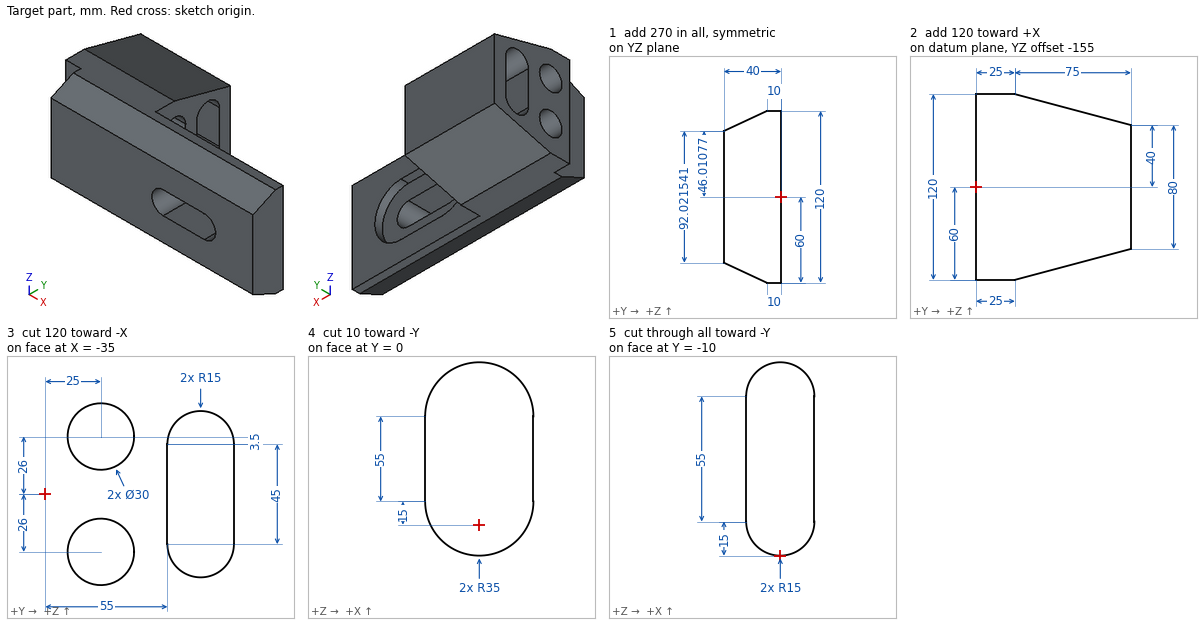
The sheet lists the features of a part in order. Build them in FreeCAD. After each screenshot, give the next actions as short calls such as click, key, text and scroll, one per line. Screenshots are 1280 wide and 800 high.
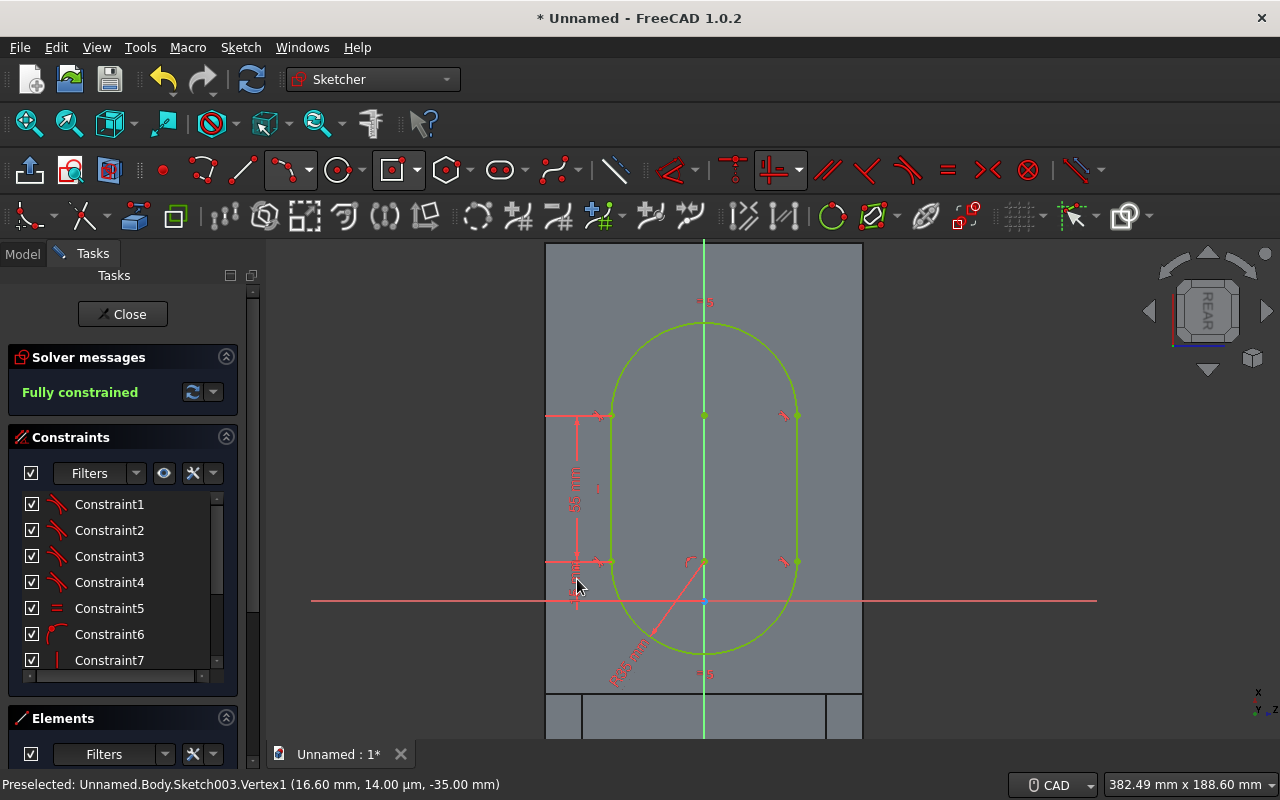
click(123, 314)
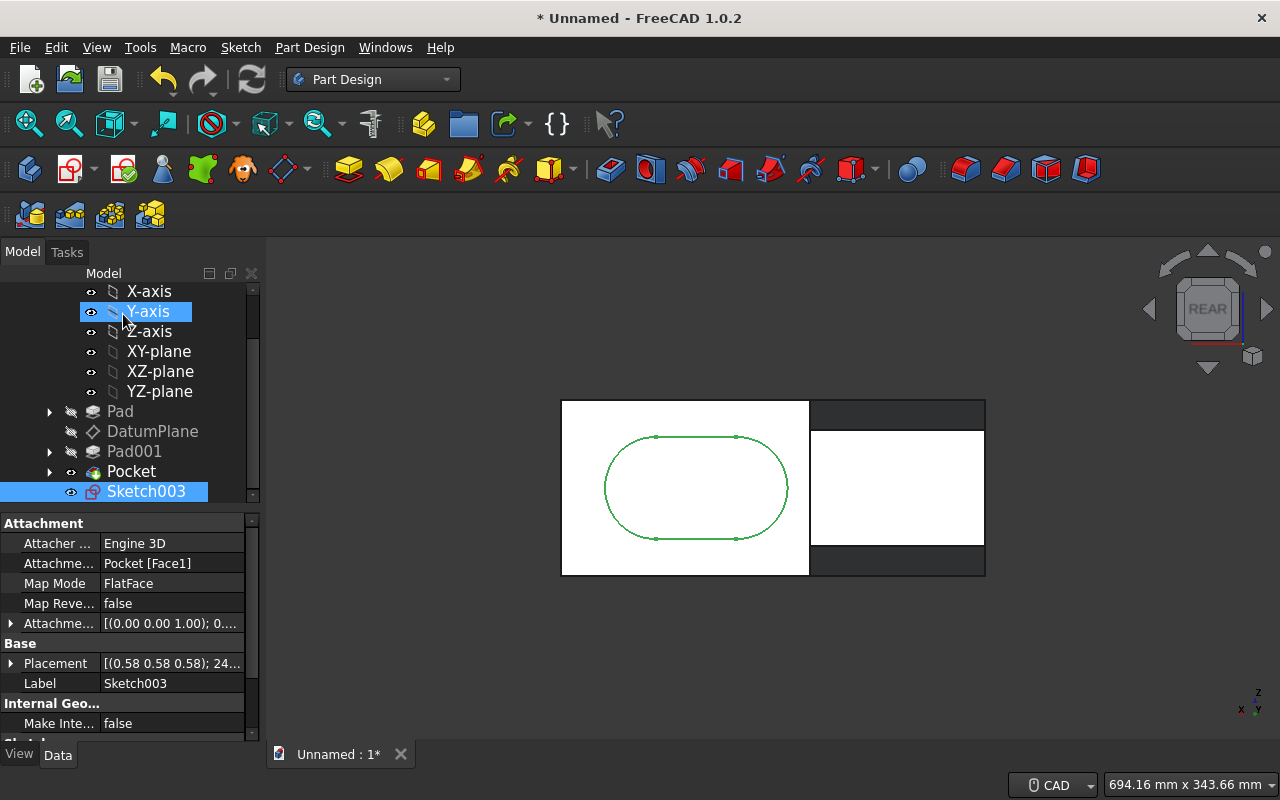
click(612, 170)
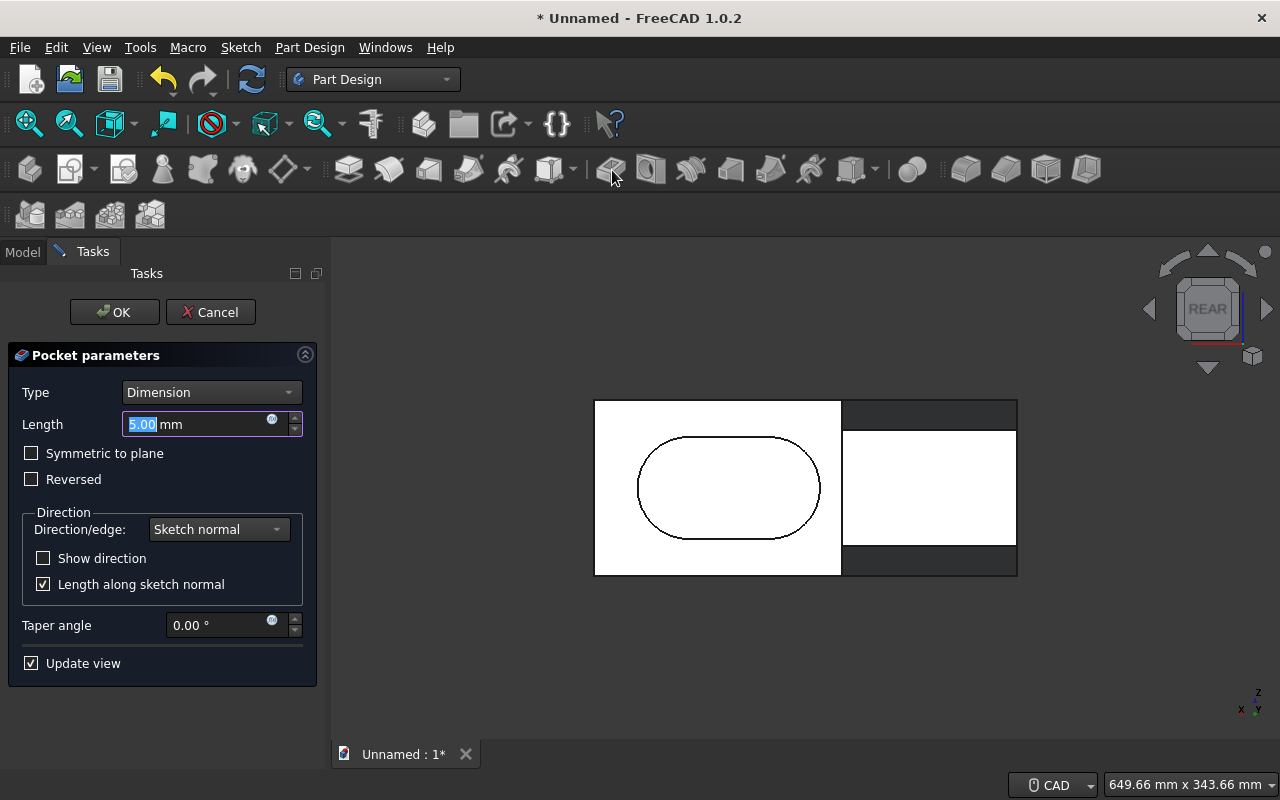
text(10)
key(Tab)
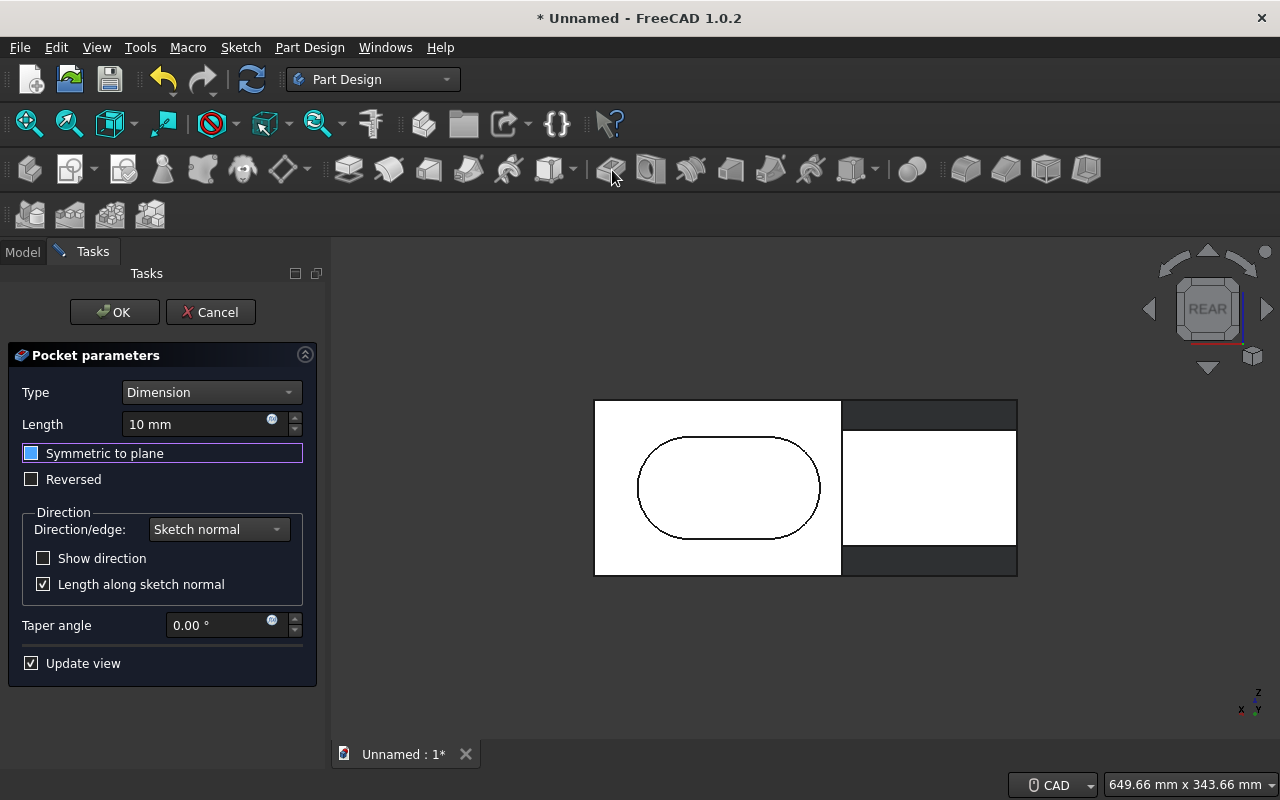
click(115, 312)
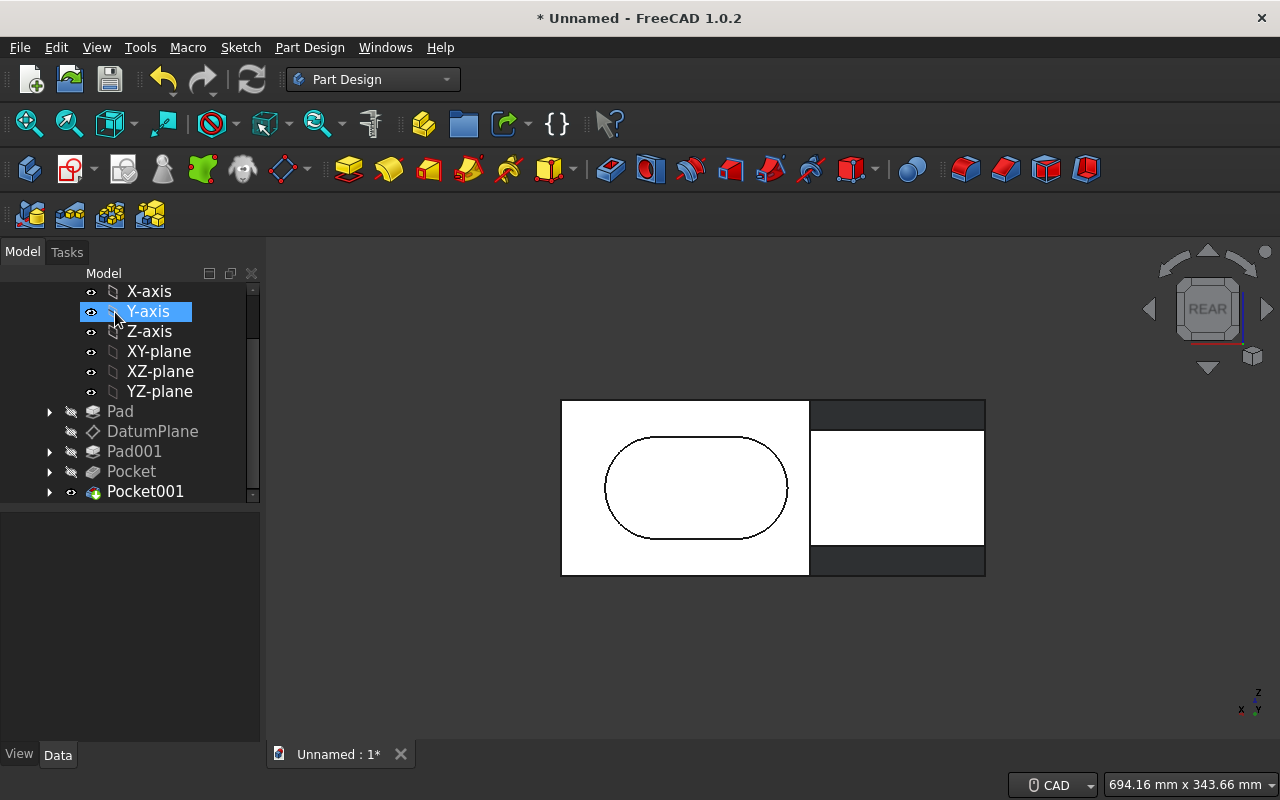
click(30, 124)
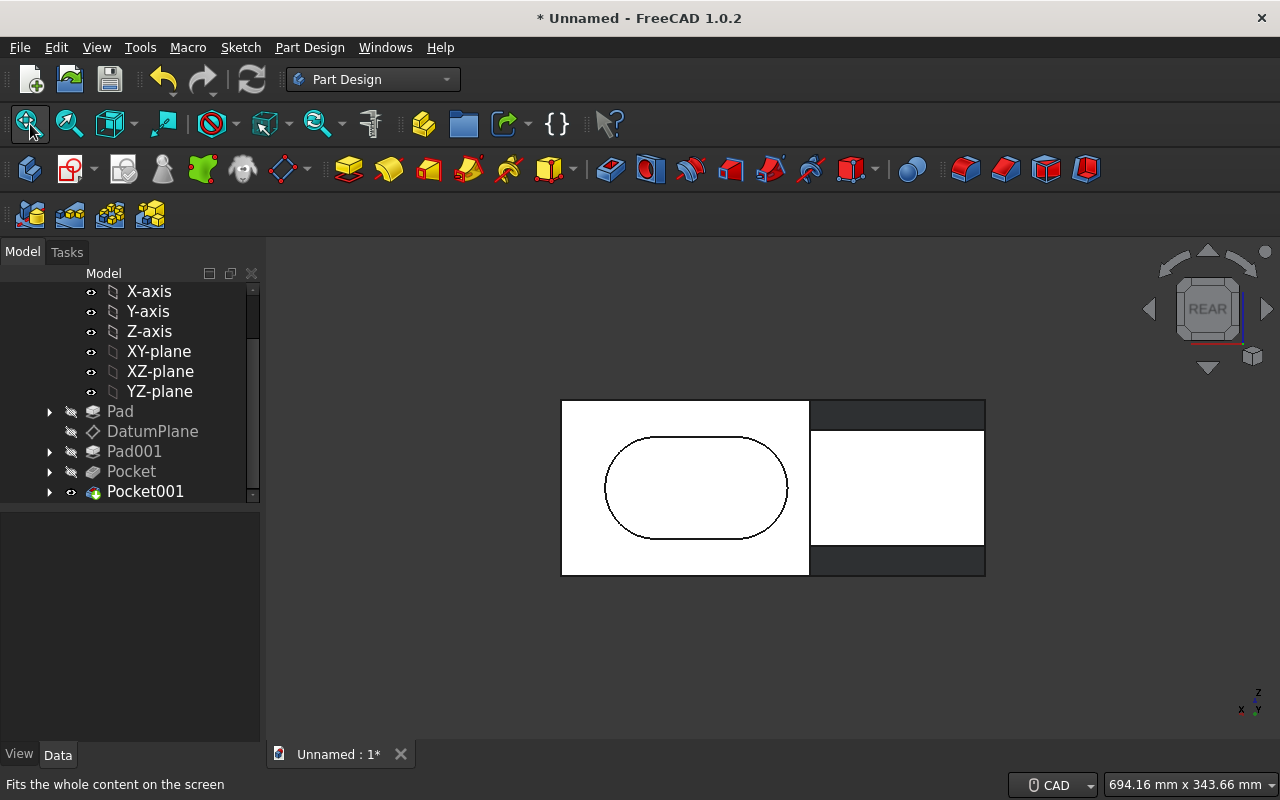
click(670, 487)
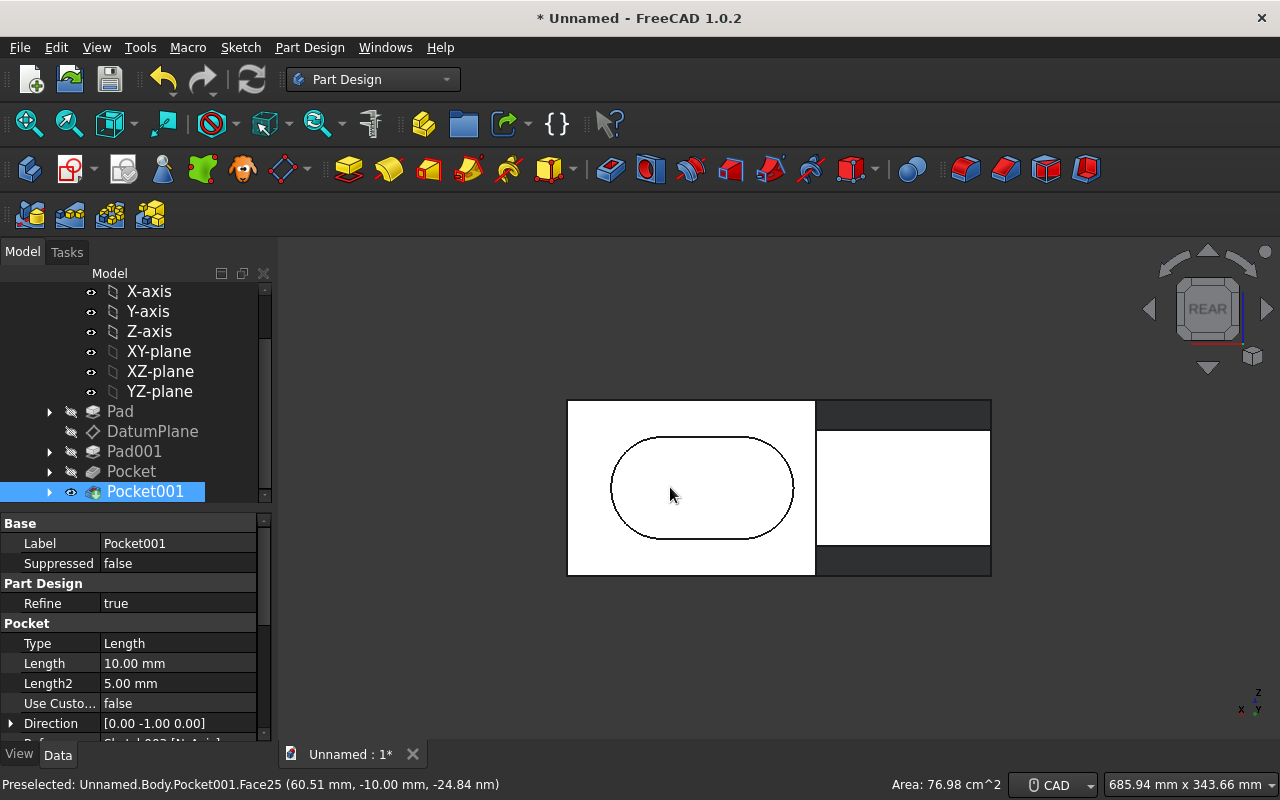
click(70, 170)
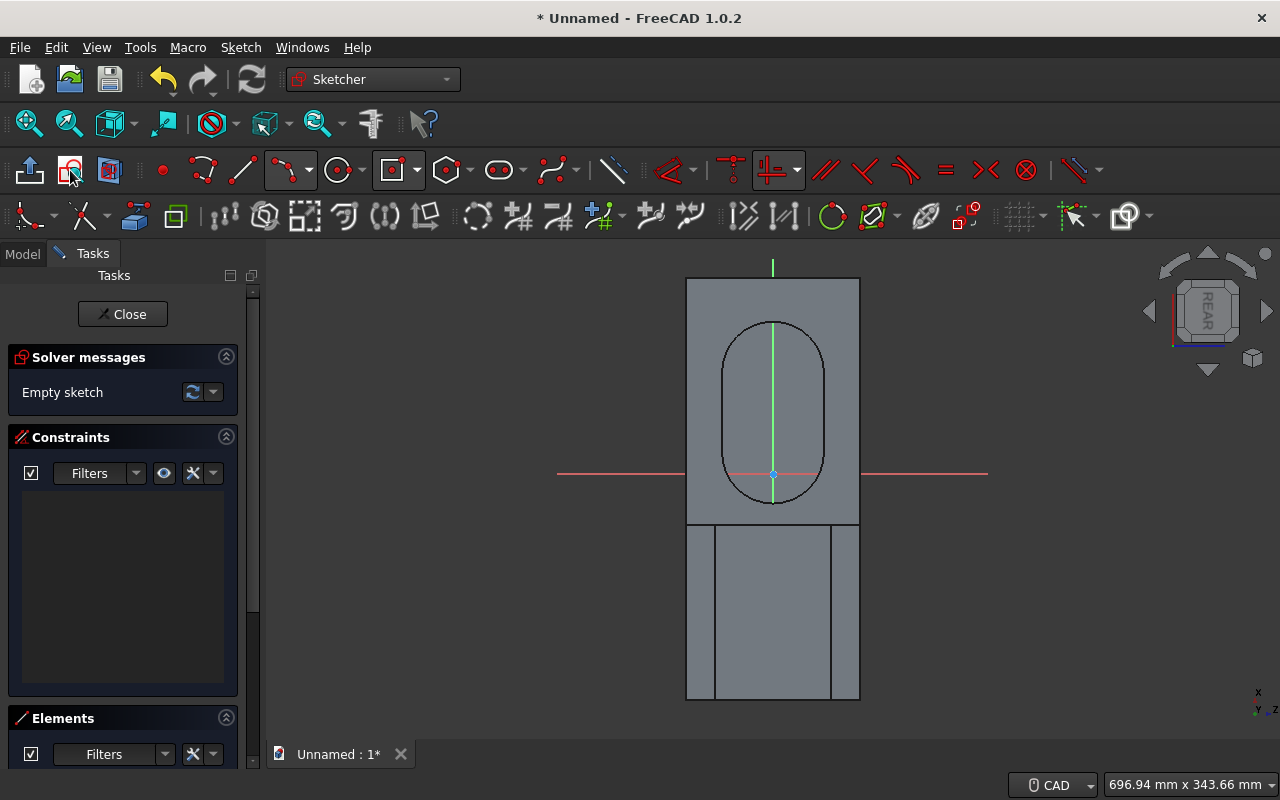
click(110, 170)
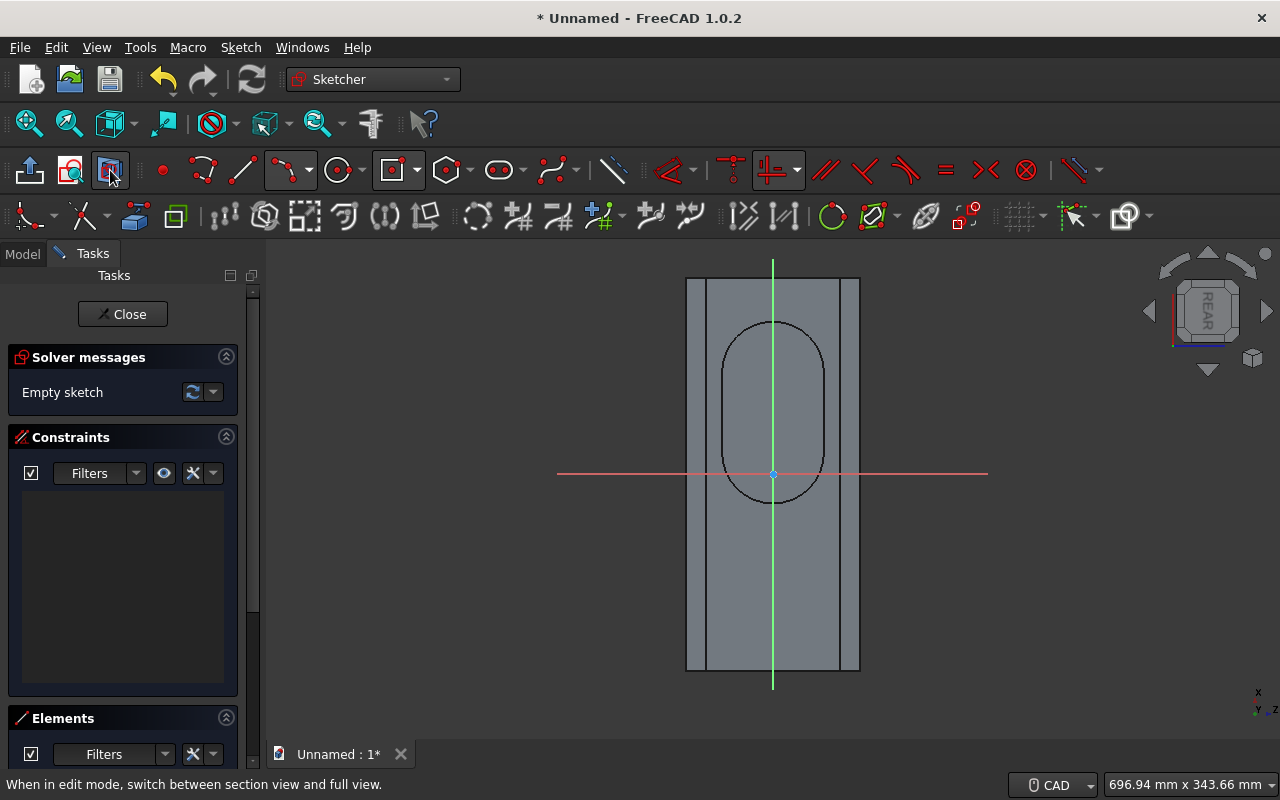
scroll(813, 368, up, 5)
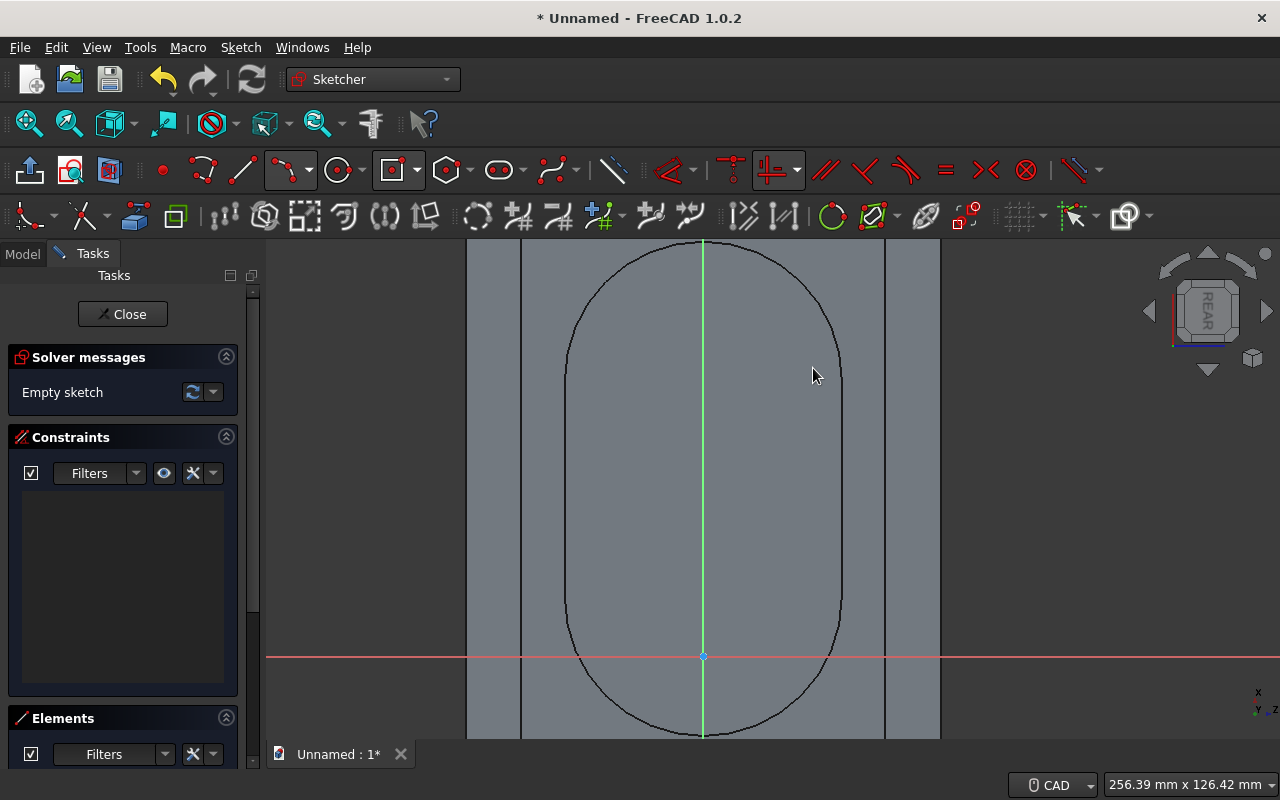
click(500, 170)